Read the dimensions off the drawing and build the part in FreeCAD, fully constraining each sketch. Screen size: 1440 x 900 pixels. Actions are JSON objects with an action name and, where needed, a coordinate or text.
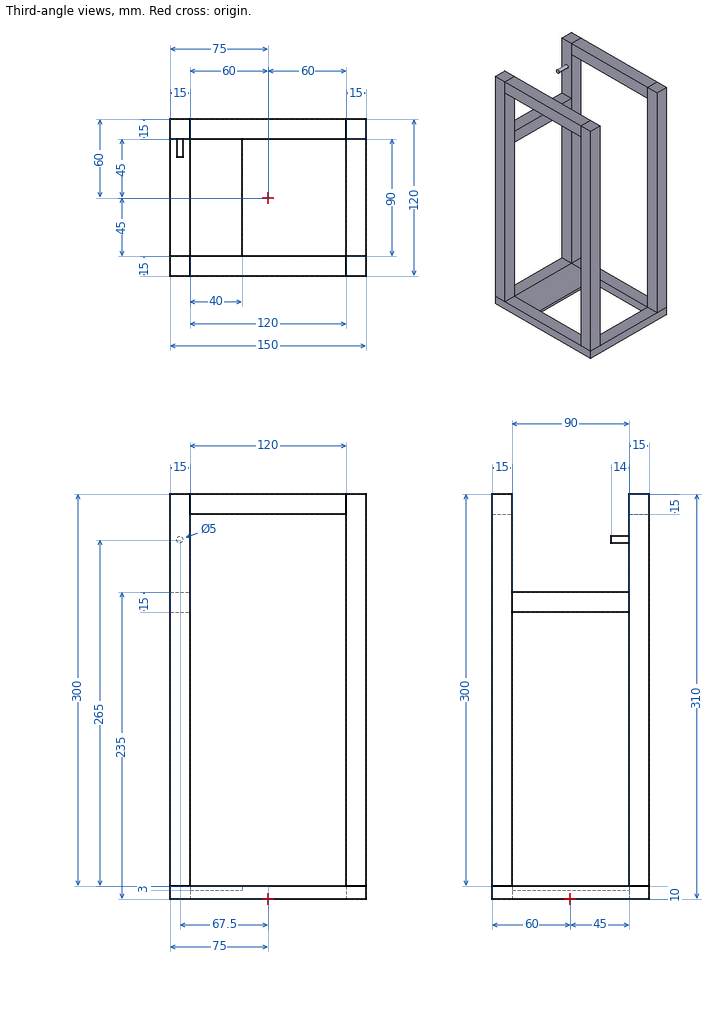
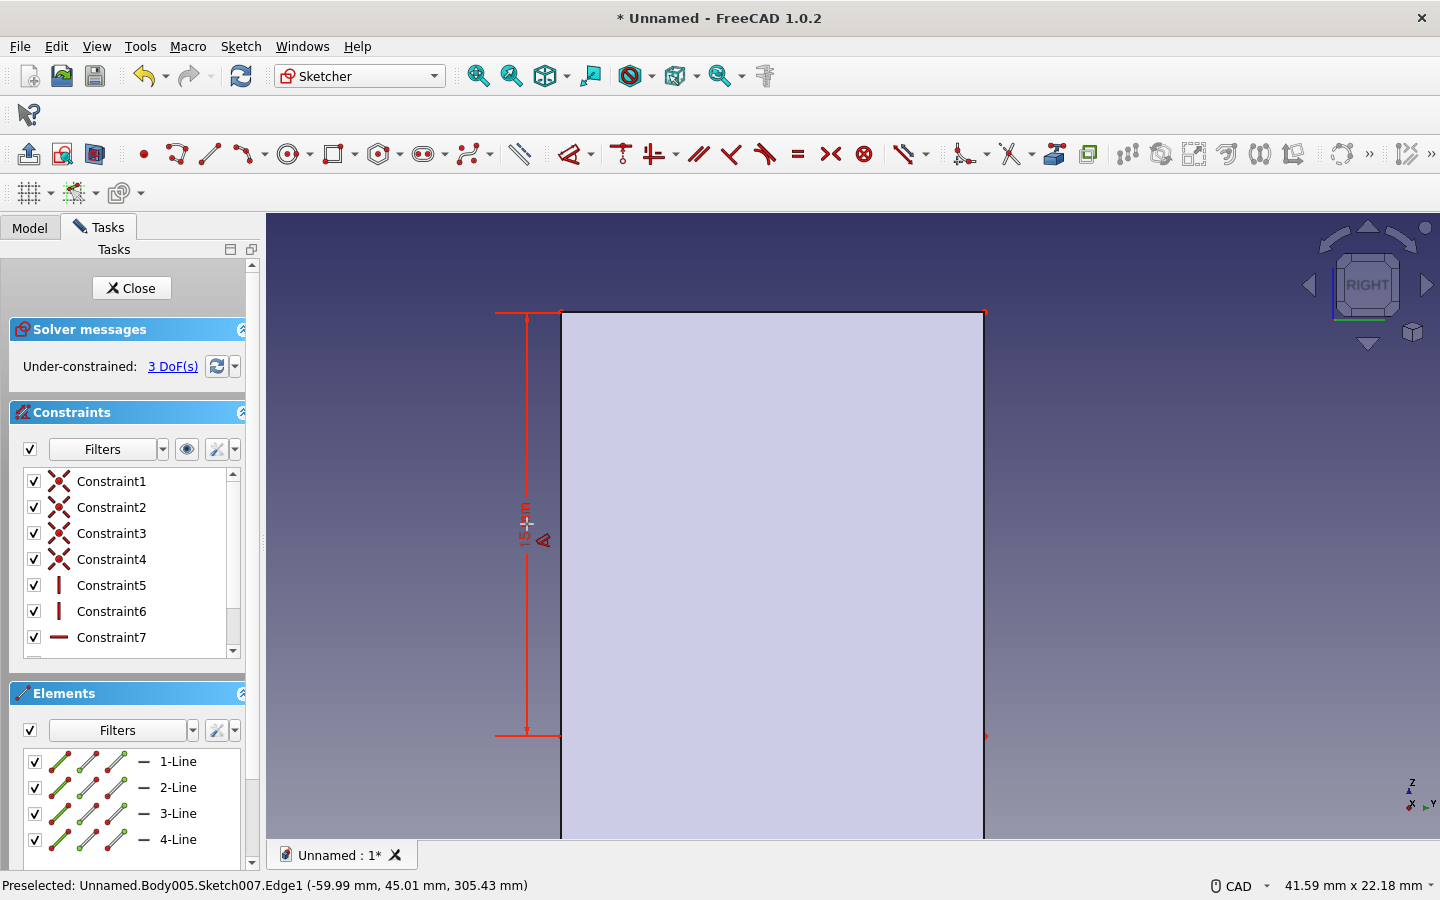
{"action": "left_click", "coordinate": [688, 736]}
{"action": "left_click", "coordinate": [772, 770]}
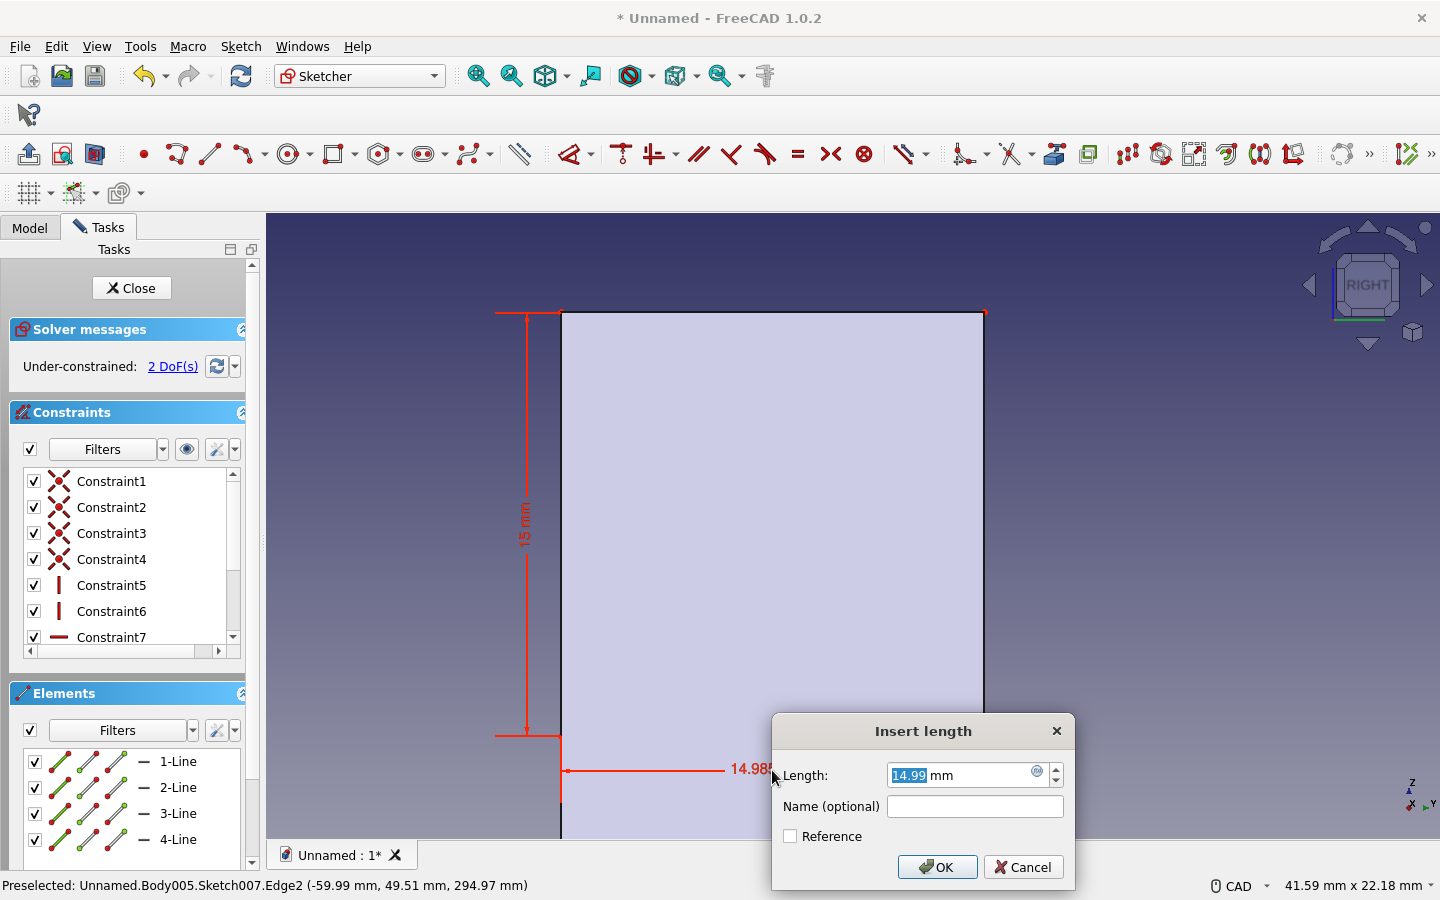
{"action": "type", "text": "15"}
{"action": "key", "text": "Return"}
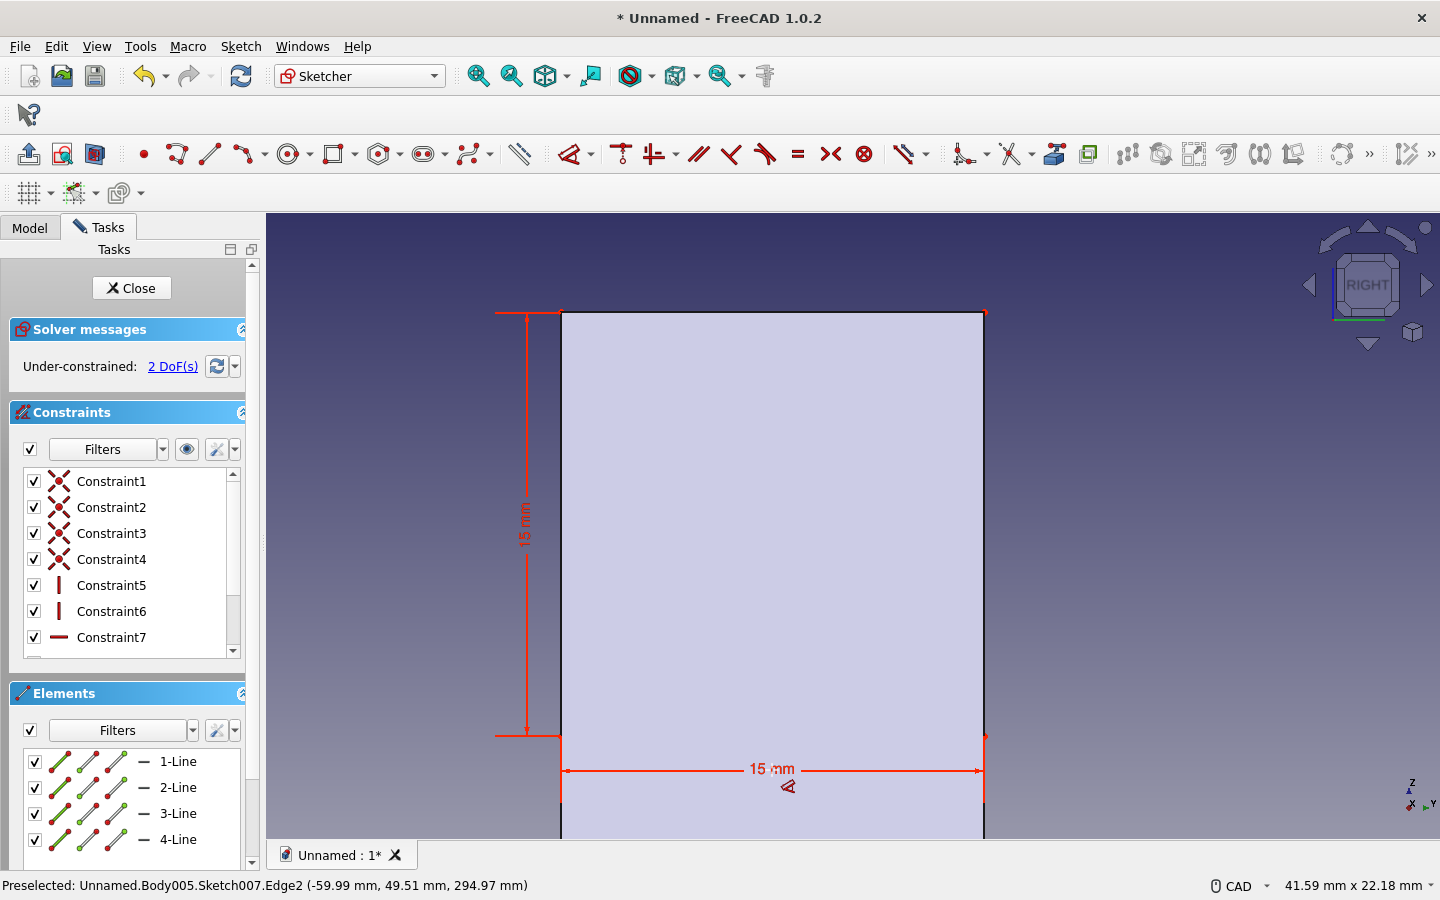
{"action": "left_click", "coordinate": [561, 313]}
{"action": "left_click", "coordinate": [428, 279]}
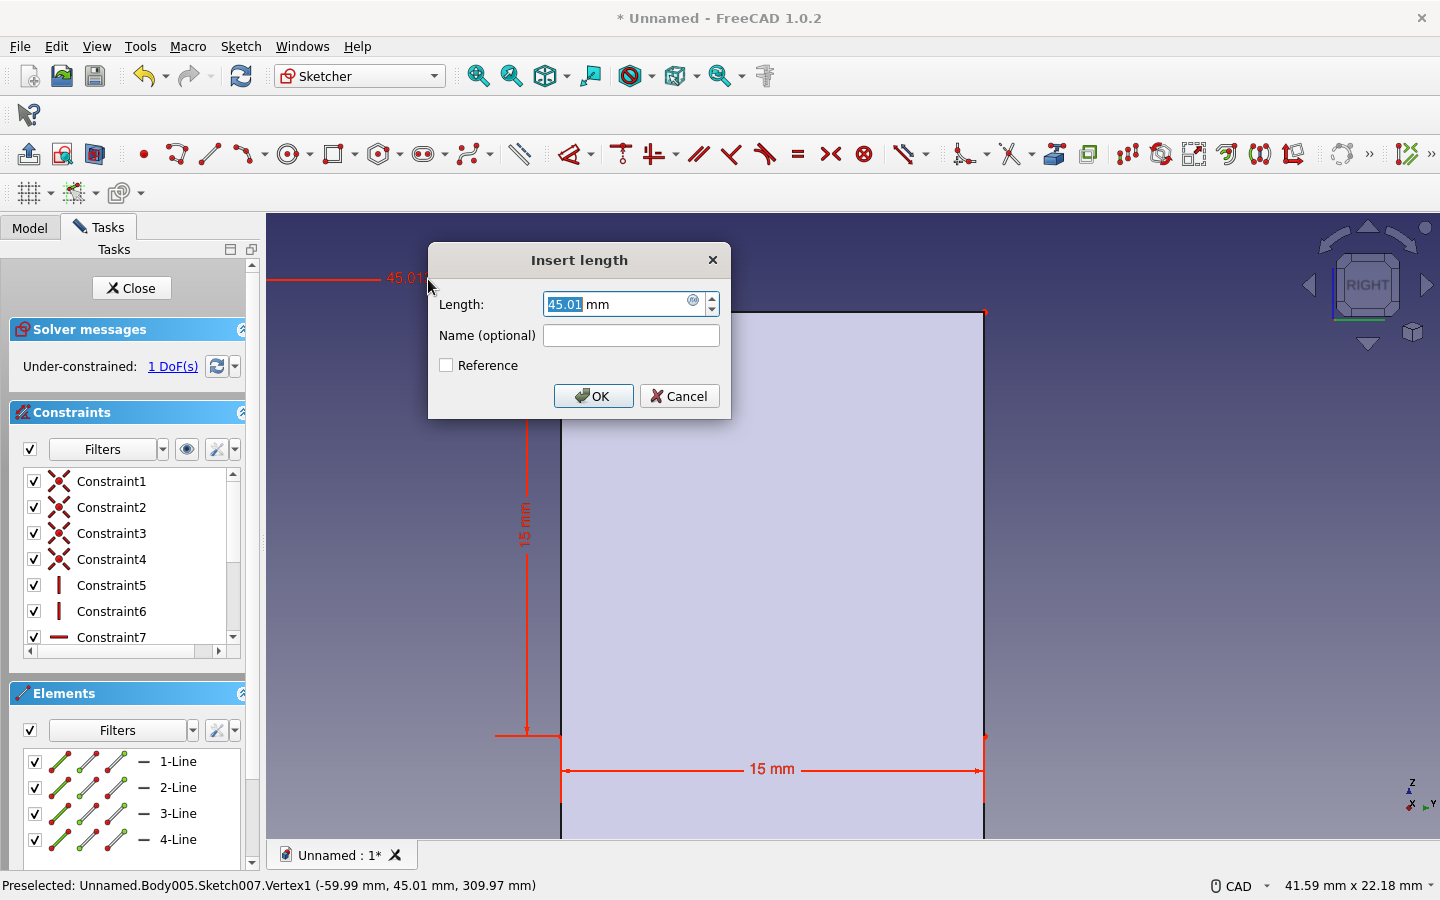
{"action": "type", "text": "45"}
{"action": "key", "text": "Return"}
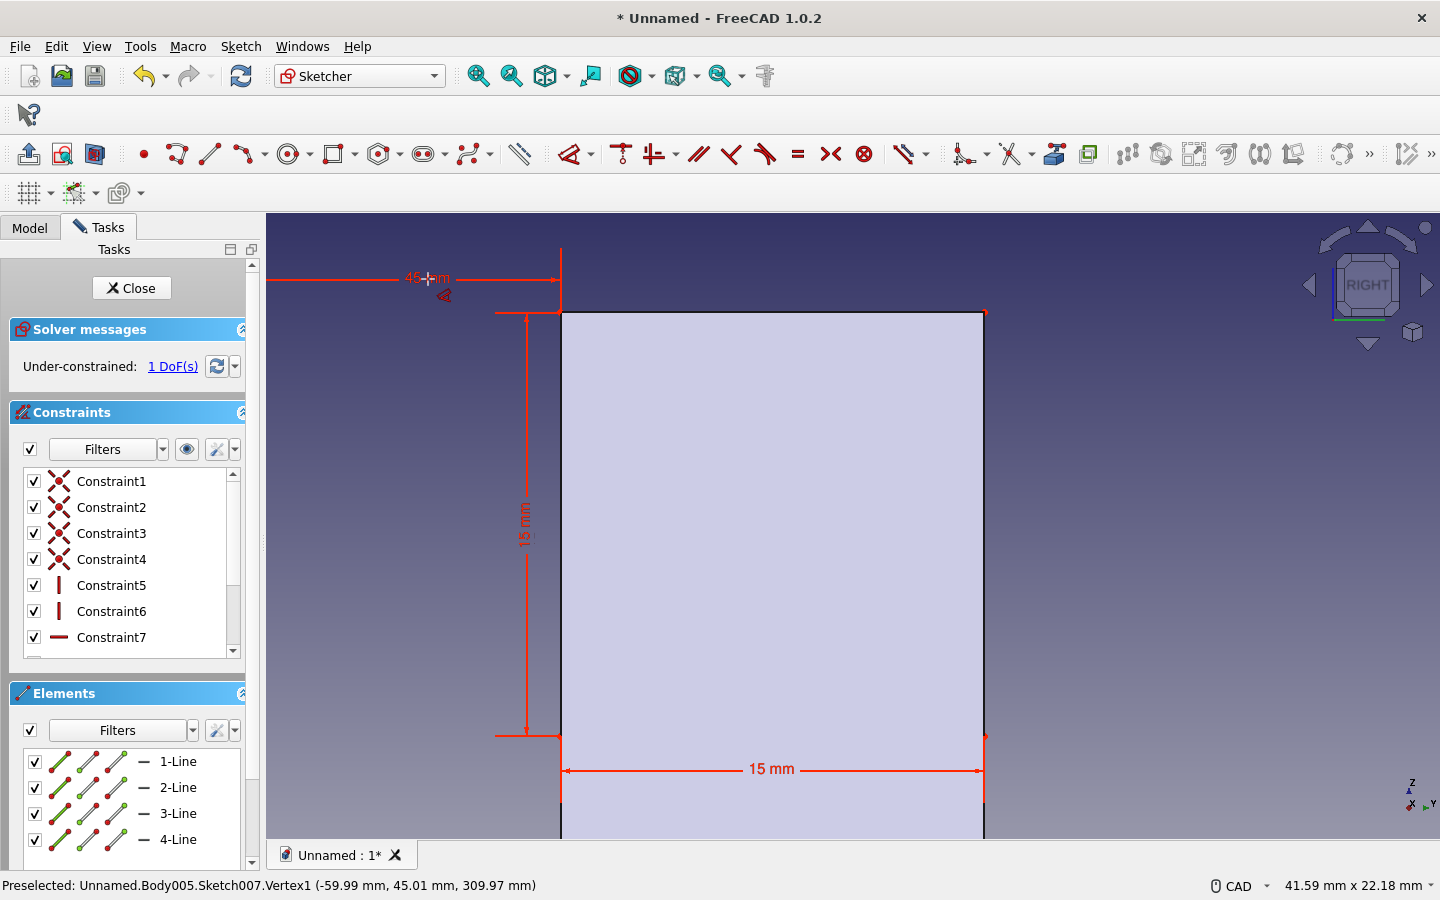
{"action": "left_click", "coordinate": [561, 313]}
{"action": "left_click", "coordinate": [595, 562]}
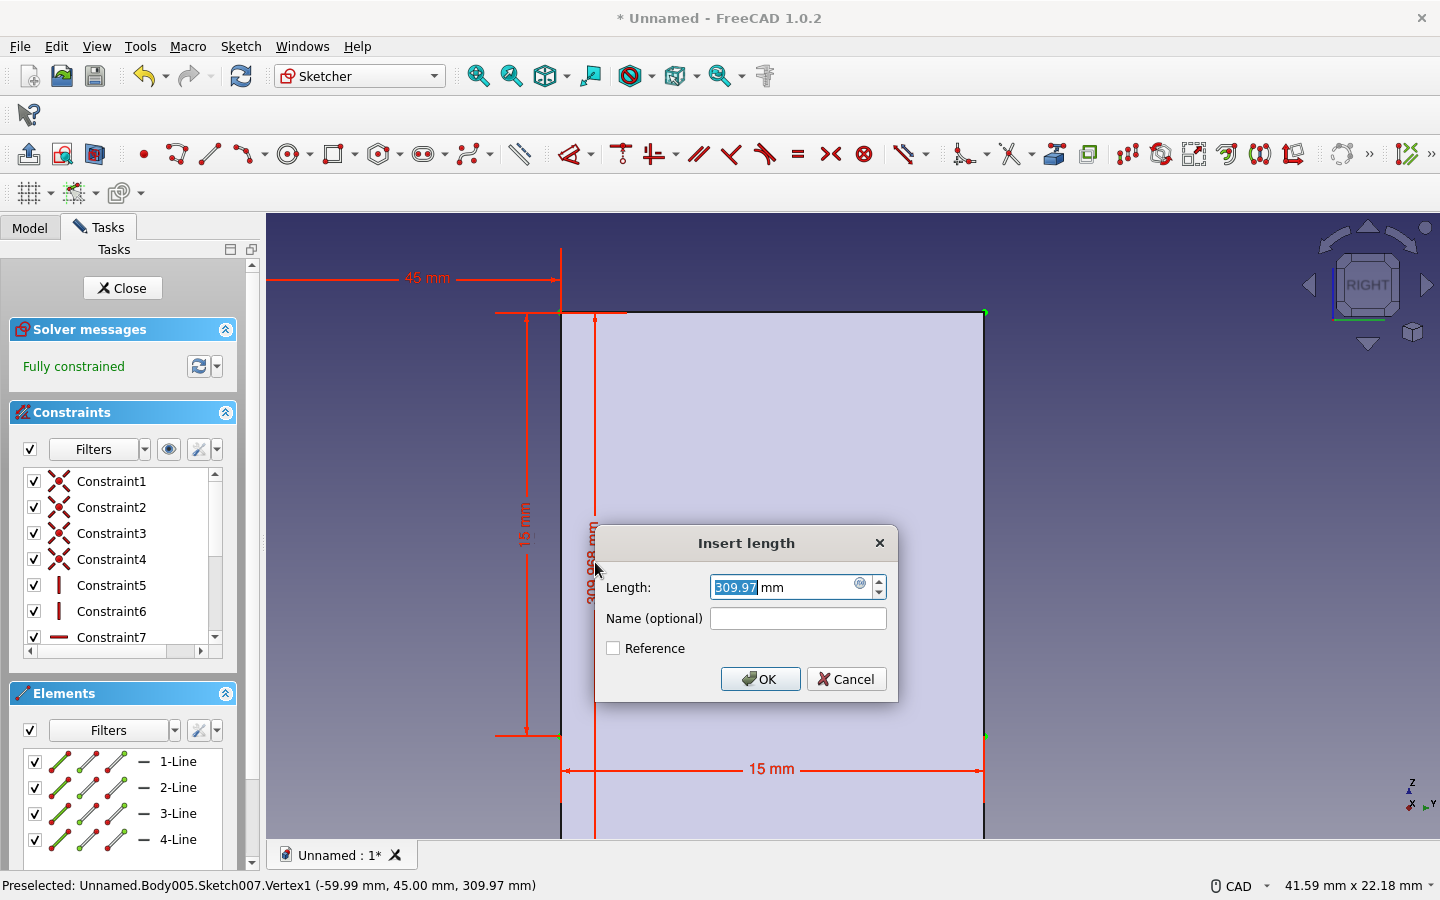
{"action": "type", "text": "310"}
{"action": "key", "text": "Return"}
{"action": "key", "text": "Escape"}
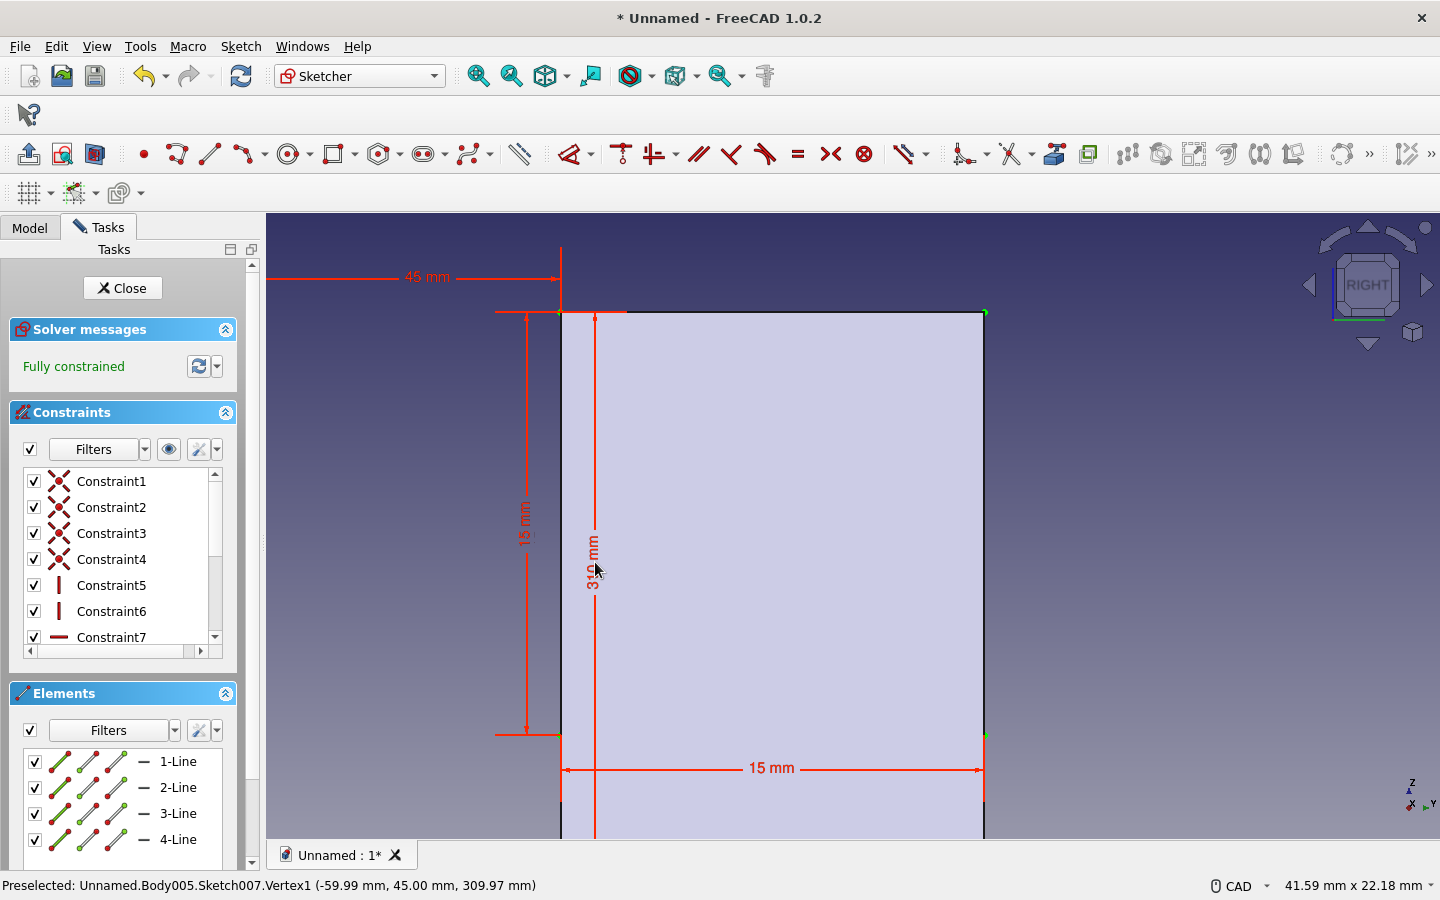
{"action": "left_click", "coordinate": [123, 288]}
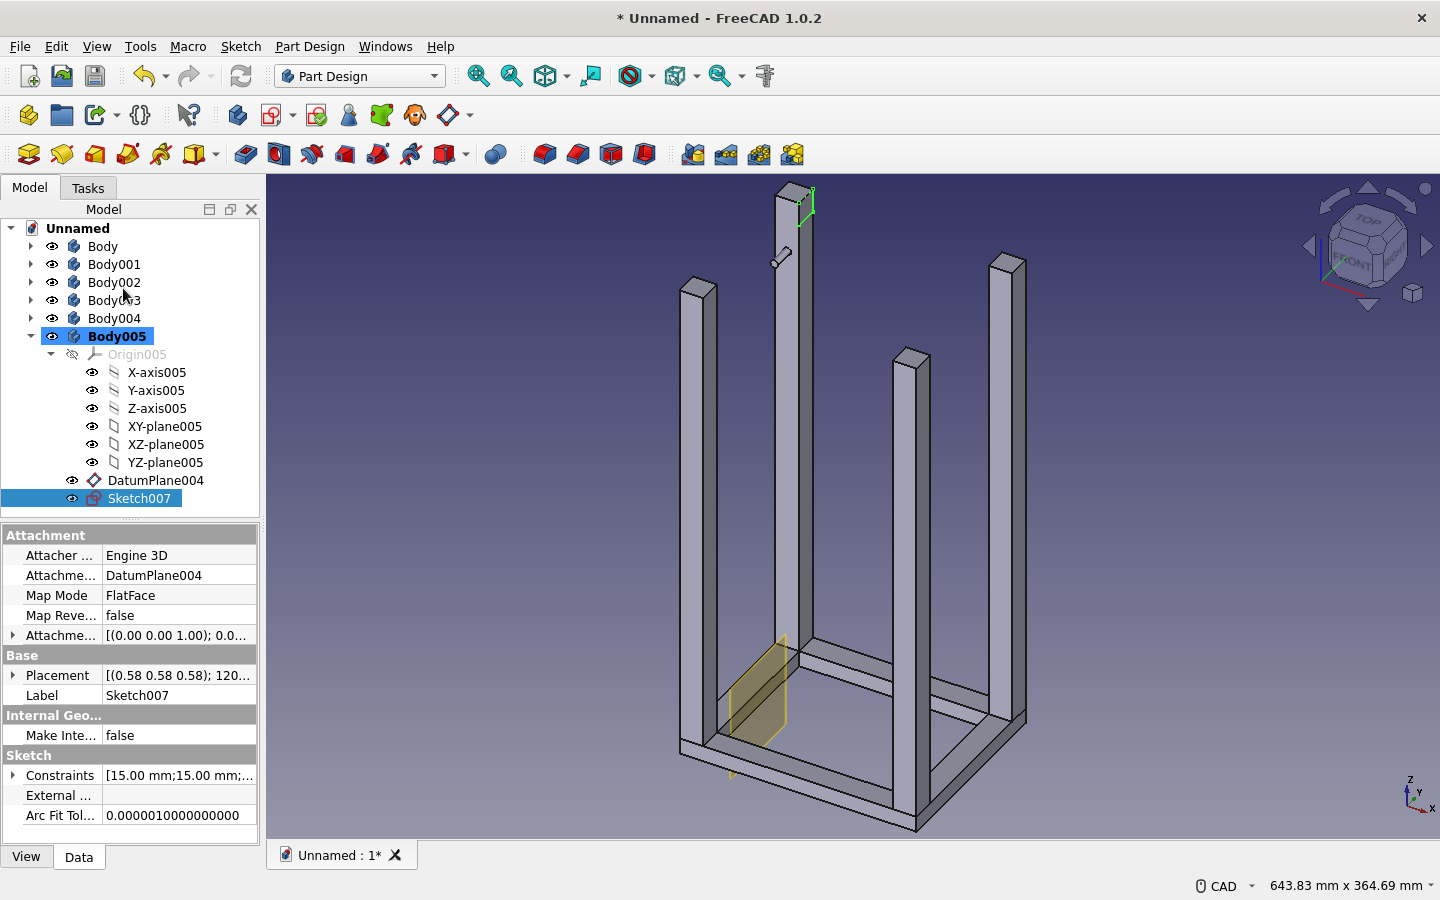
{"action": "left_click", "coordinate": [29, 154]}